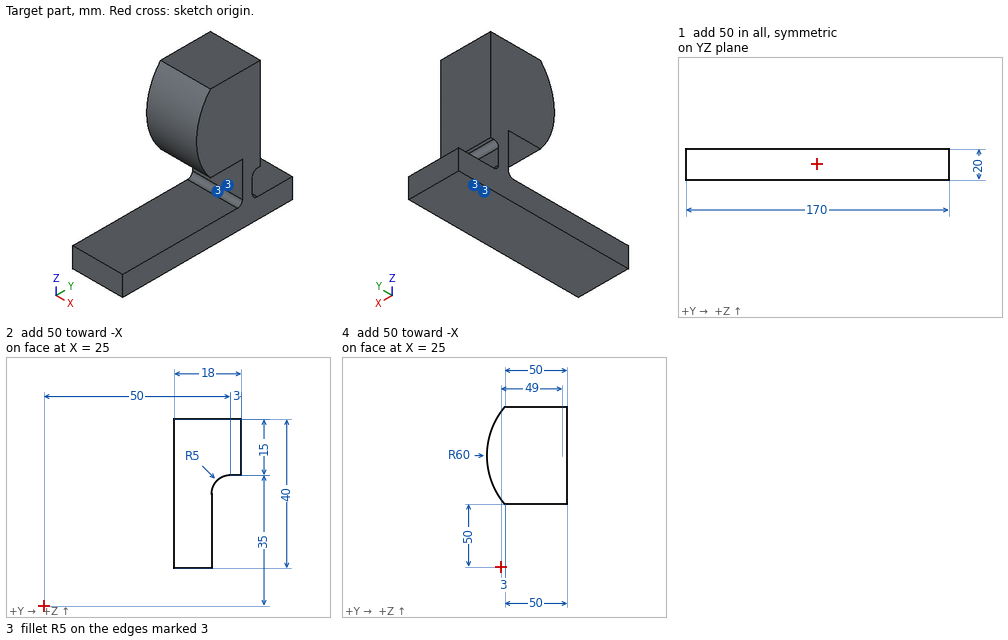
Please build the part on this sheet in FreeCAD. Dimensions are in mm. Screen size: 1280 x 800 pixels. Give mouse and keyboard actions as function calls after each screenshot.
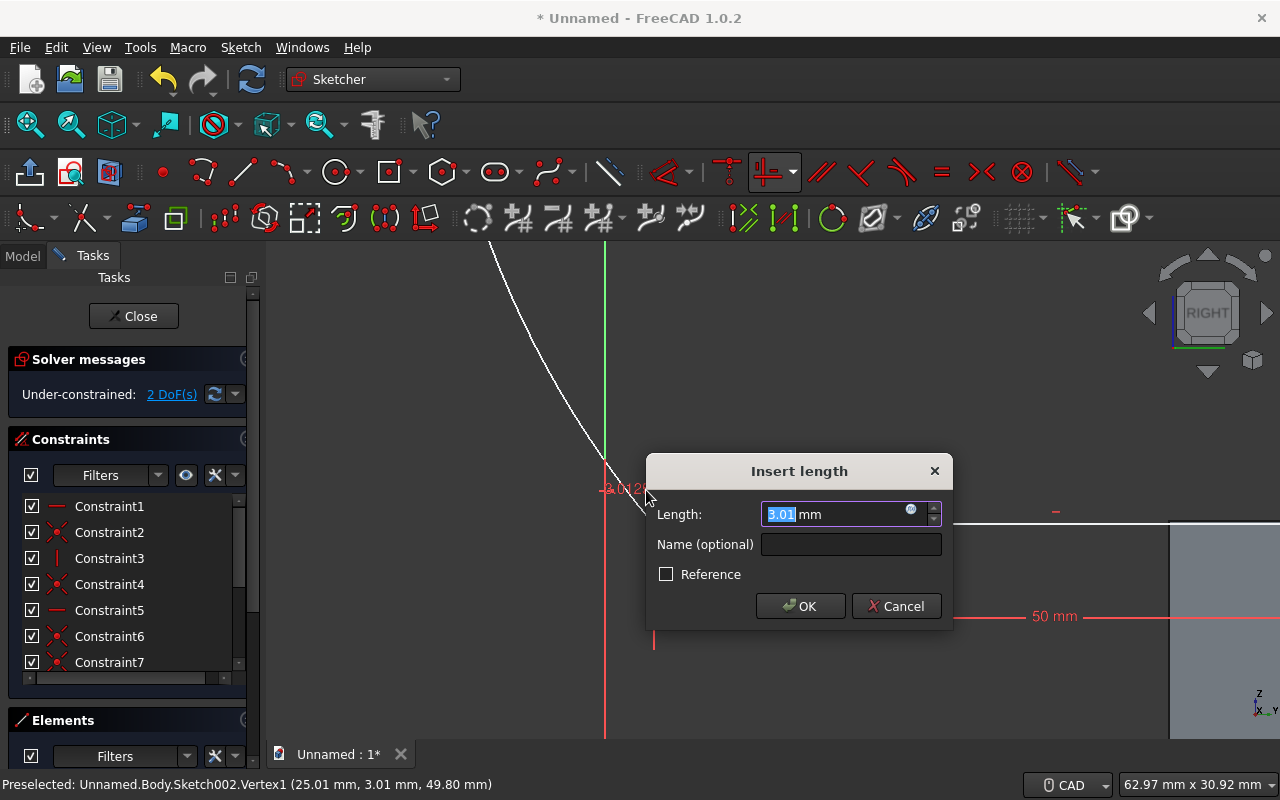
text(3)
key(Return)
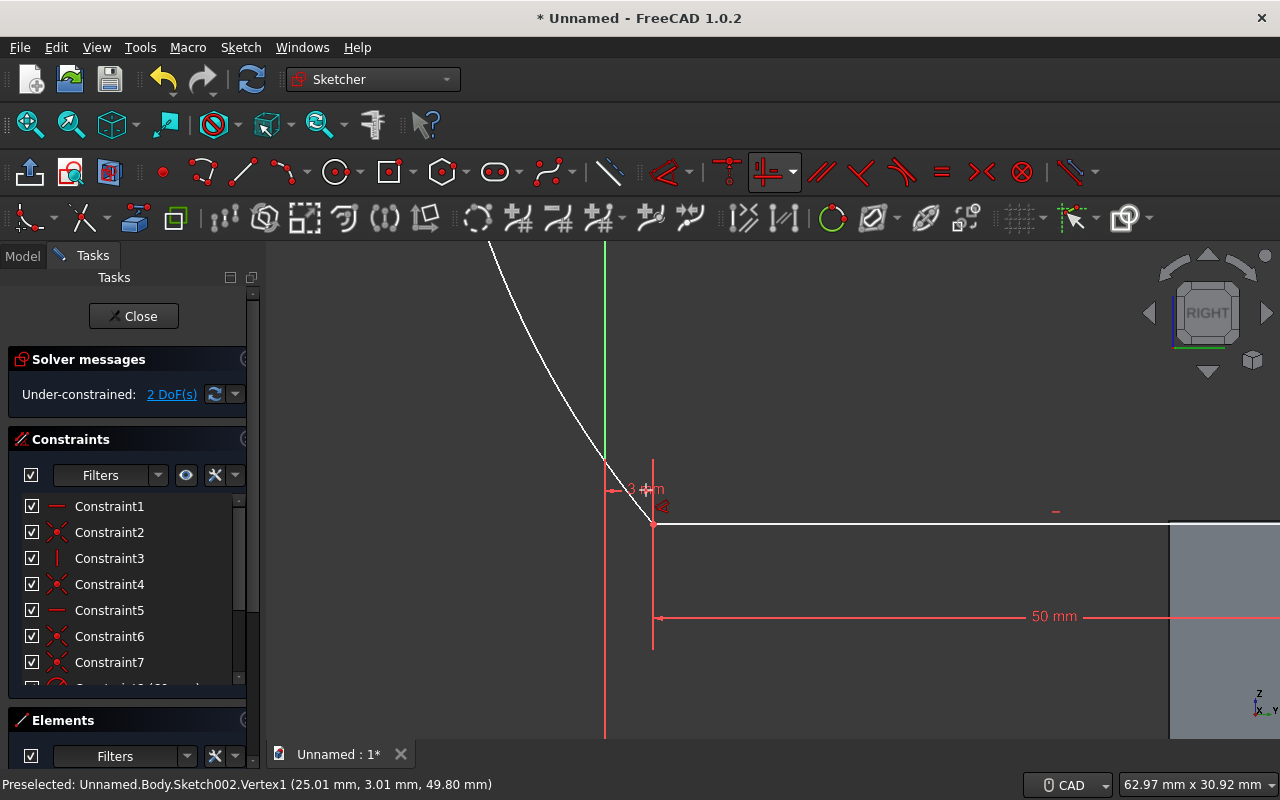
scroll(657, 527, down, 9)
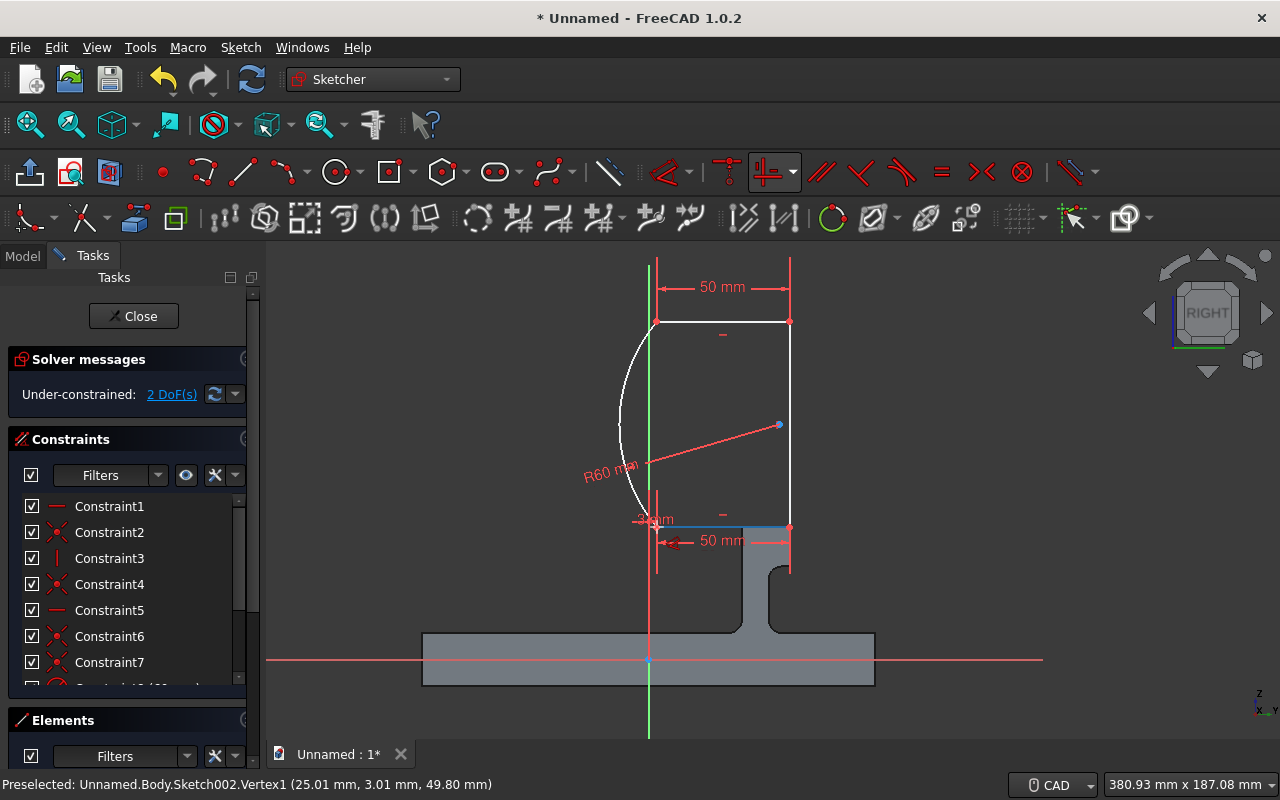
click(657, 527)
click(615, 593)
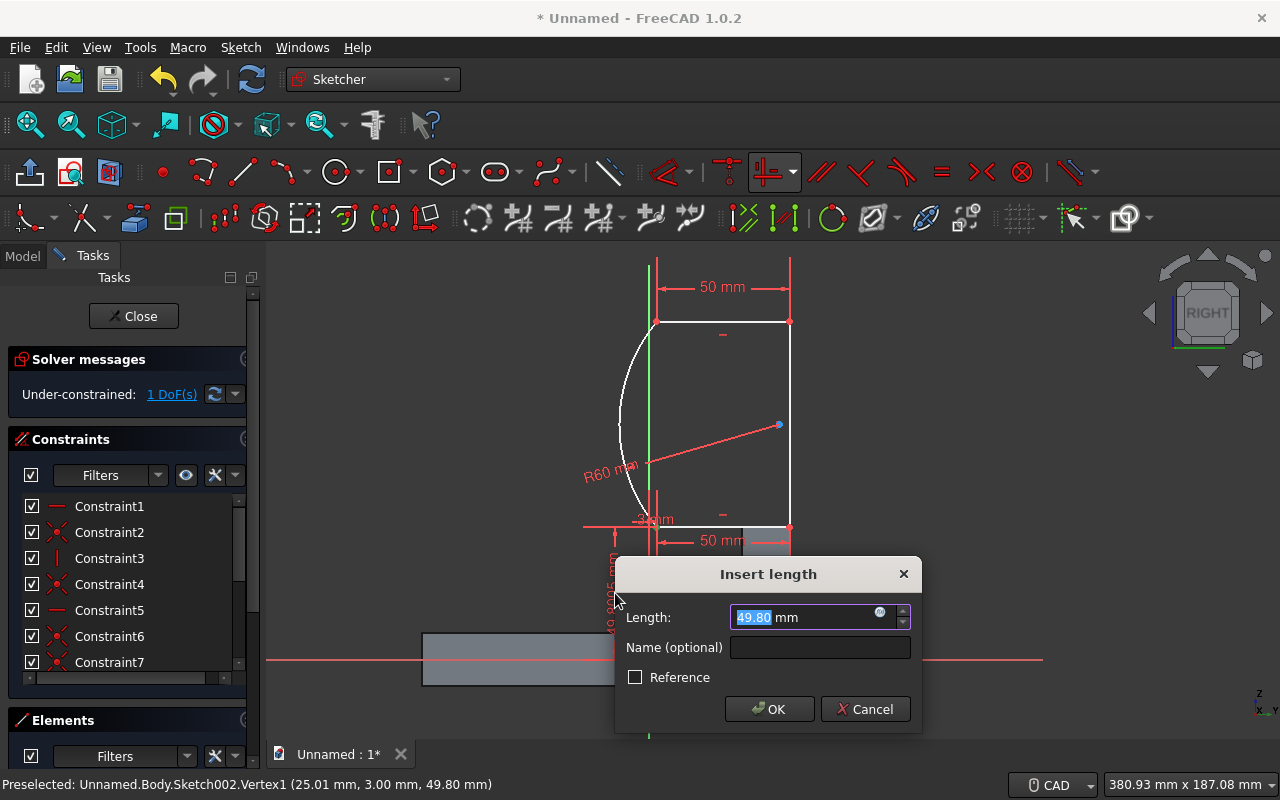
text(50)
key(Return)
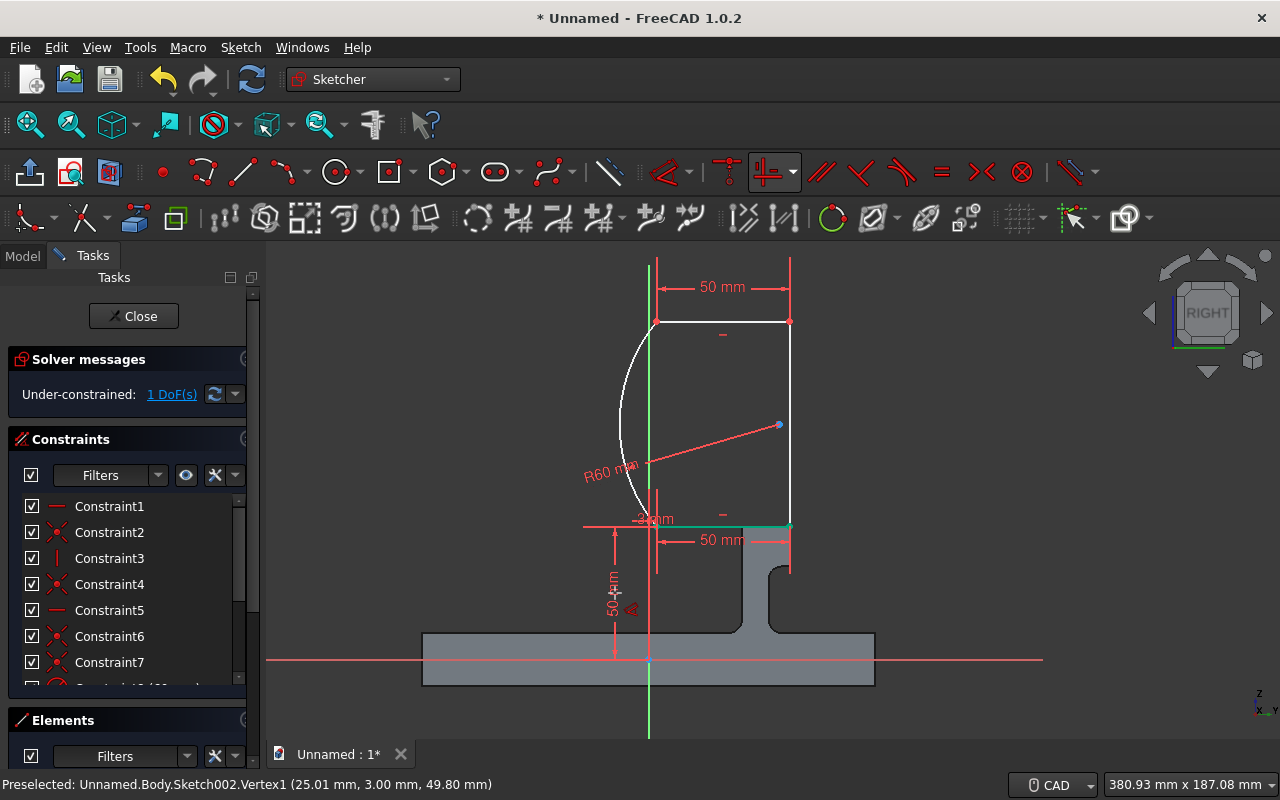
click(779, 424)
click(714, 694)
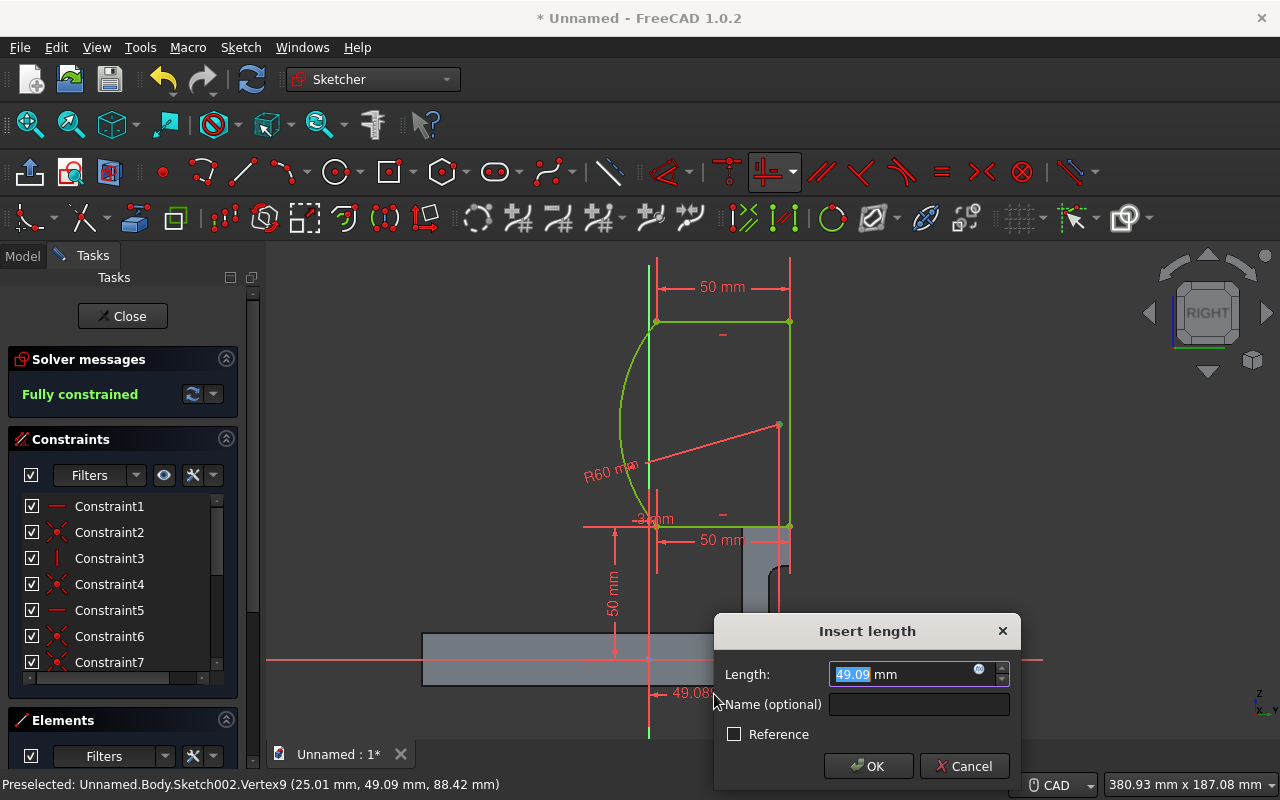
text(49)
key(Return)
key(Escape)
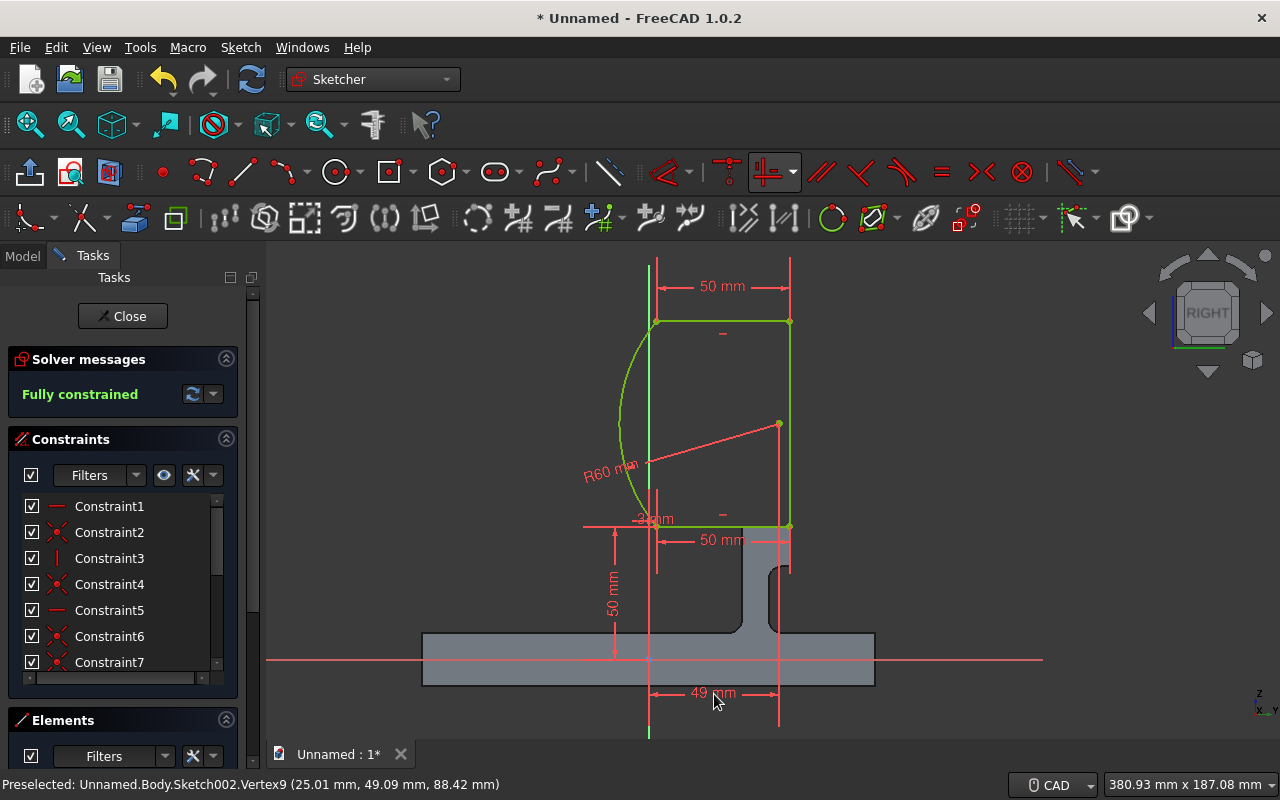
click(123, 316)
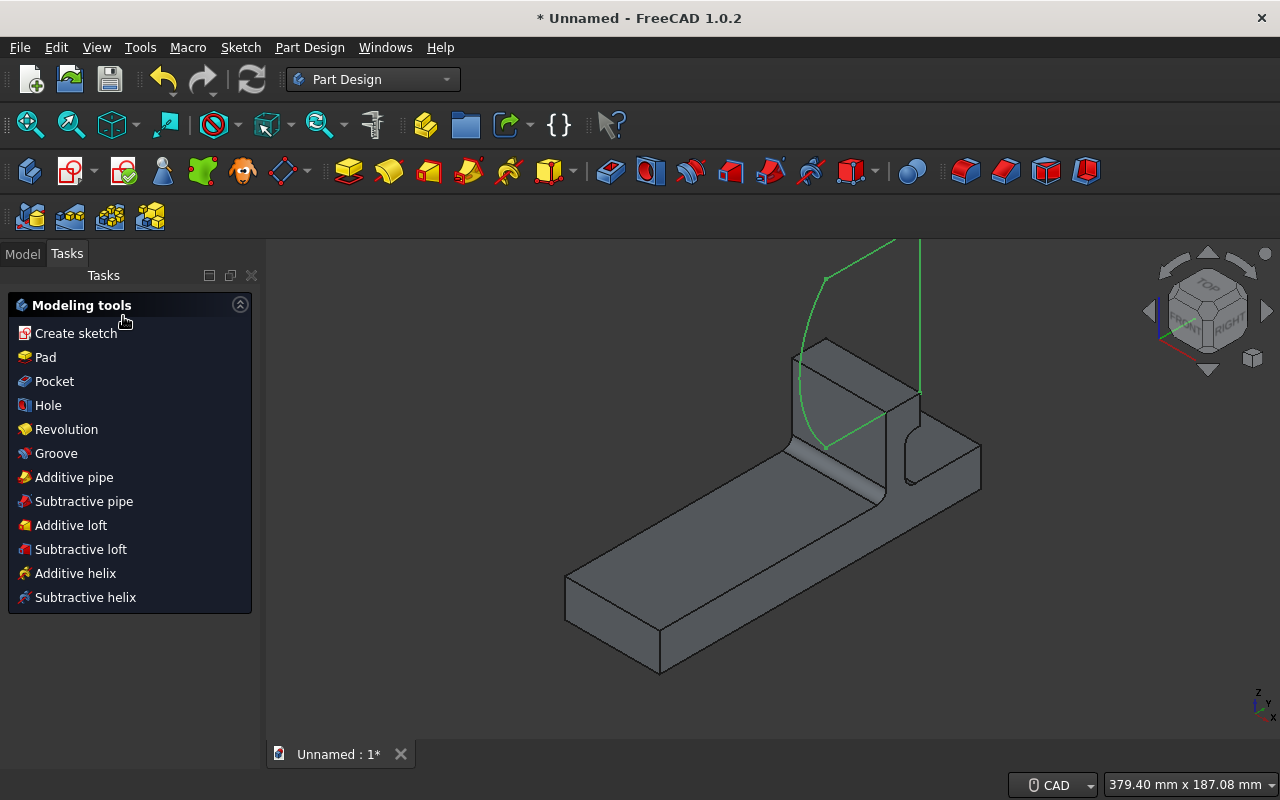
click(350, 172)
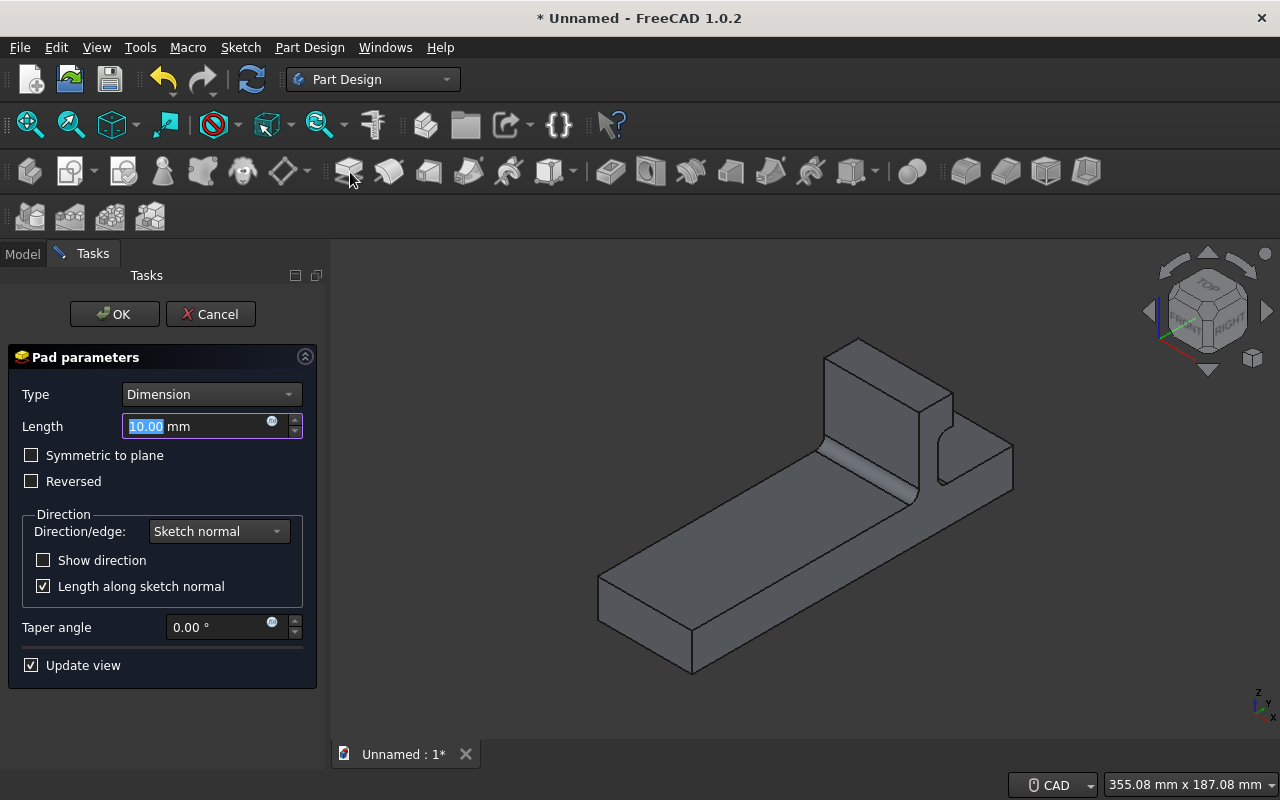
text(50)
key(Tab)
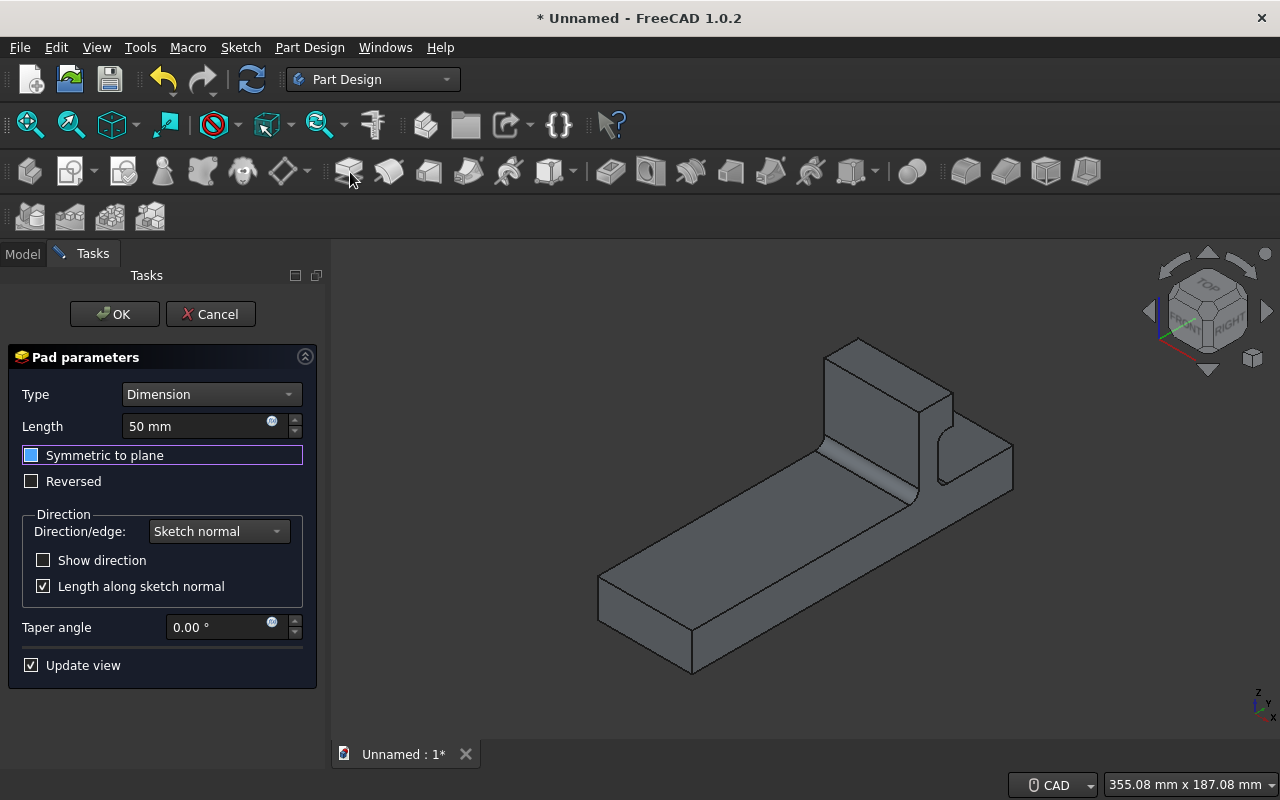
click(30, 481)